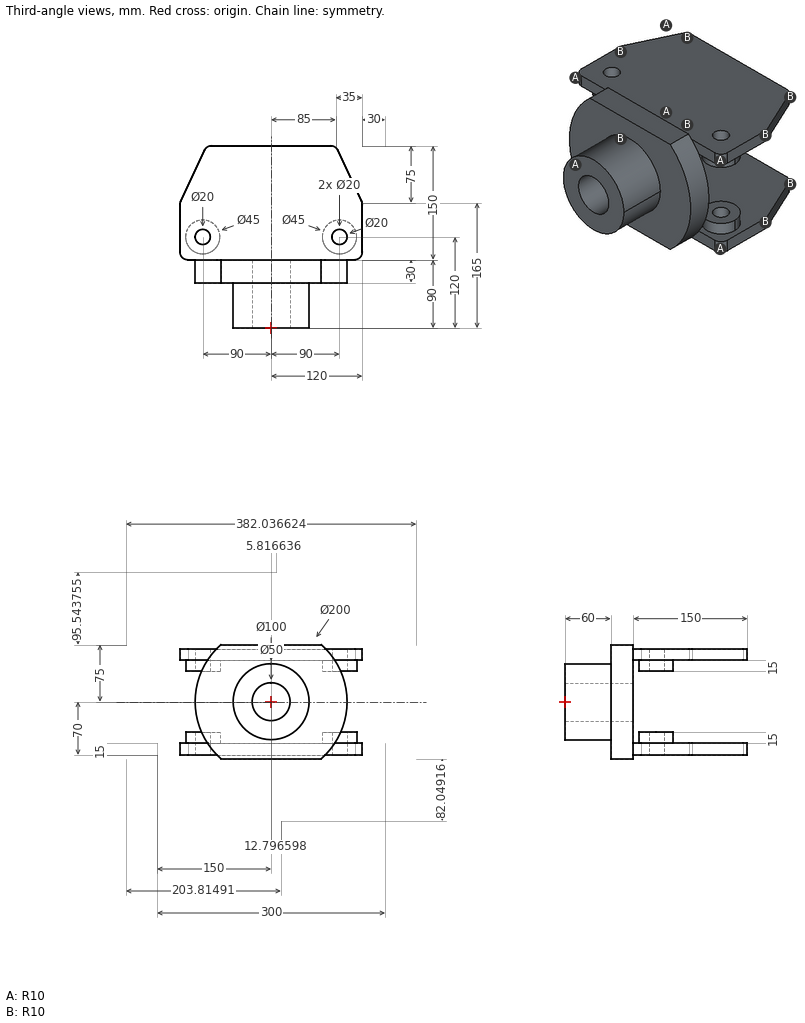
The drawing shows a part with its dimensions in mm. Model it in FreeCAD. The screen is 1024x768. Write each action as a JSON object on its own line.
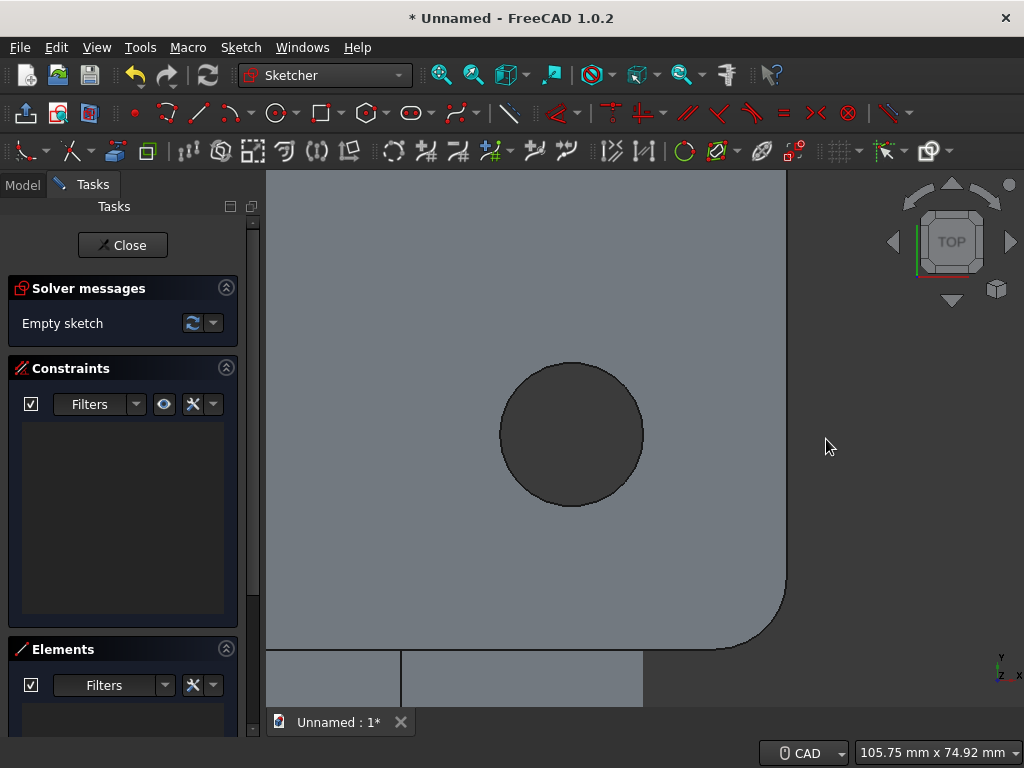
{"action": "left_click", "coordinate": [276, 114]}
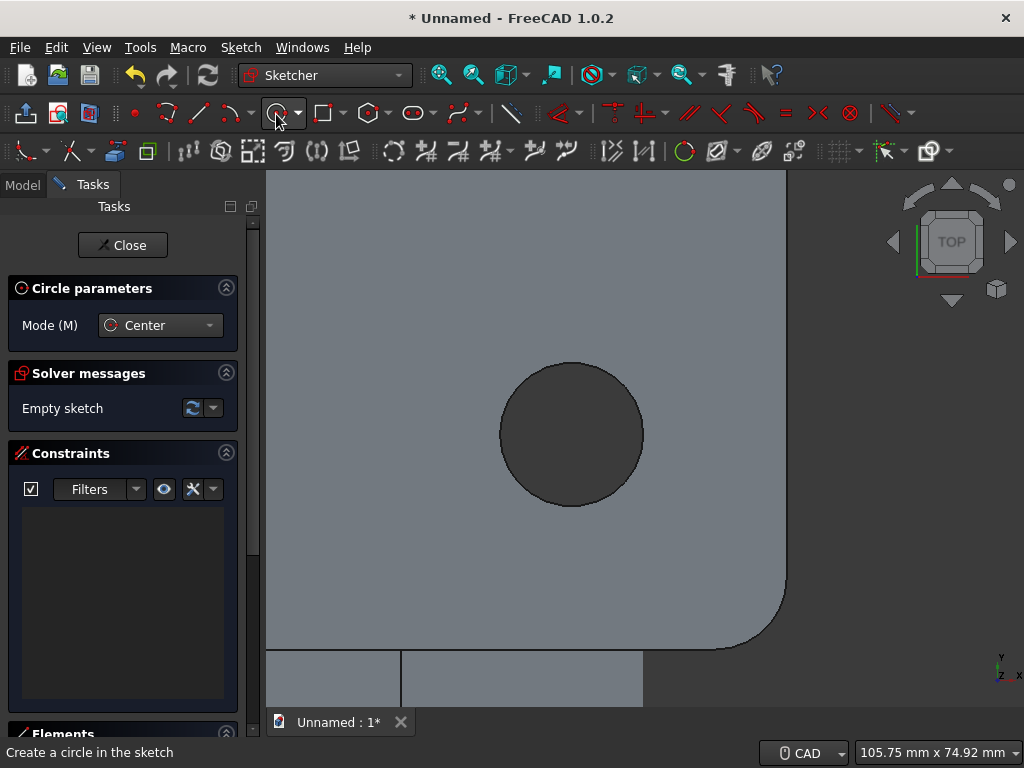
{"action": "left_click", "coordinate": [572, 435]}
{"action": "left_click", "coordinate": [686, 321]}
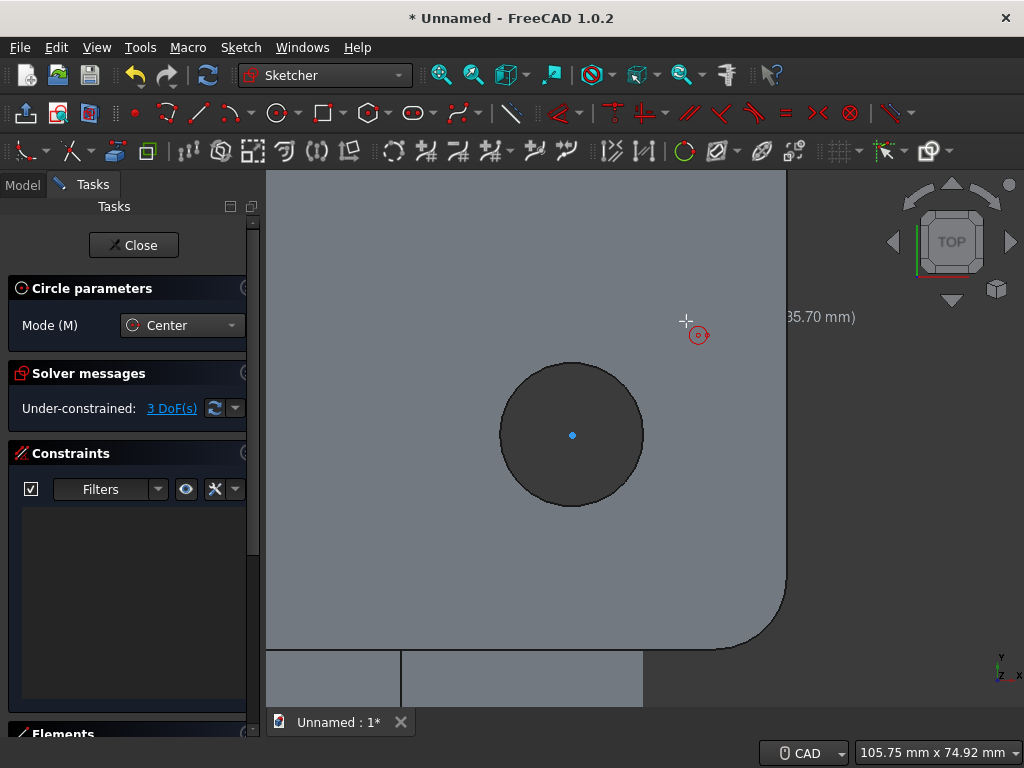
{"action": "left_click", "coordinate": [572, 436]}
{"action": "left_click", "coordinate": [622, 384]}
{"action": "key", "text": "Escape"}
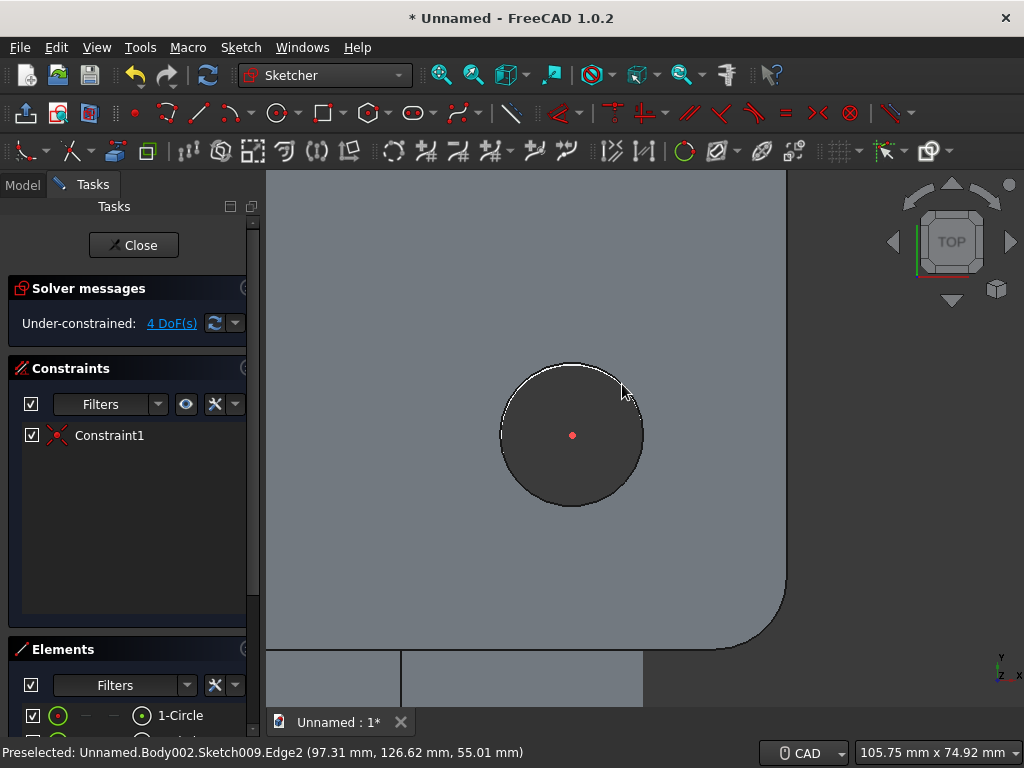
{"action": "left_click", "coordinate": [558, 114]}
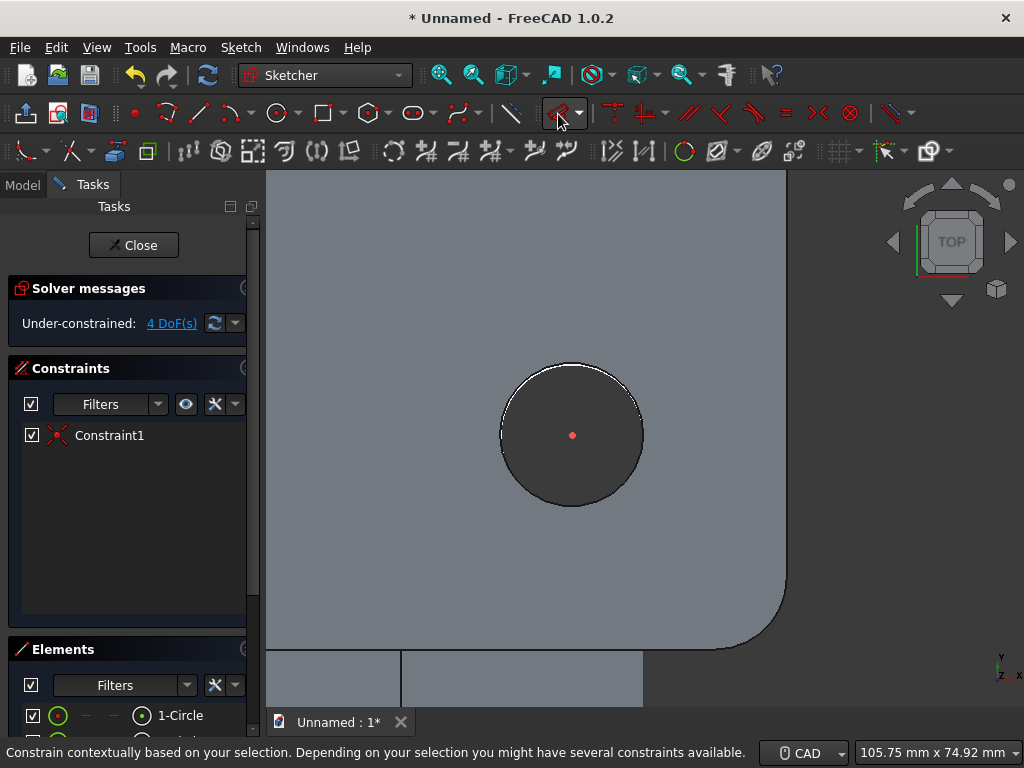
{"action": "left_click", "coordinate": [686, 322]}
{"action": "left_click", "coordinate": [709, 299]}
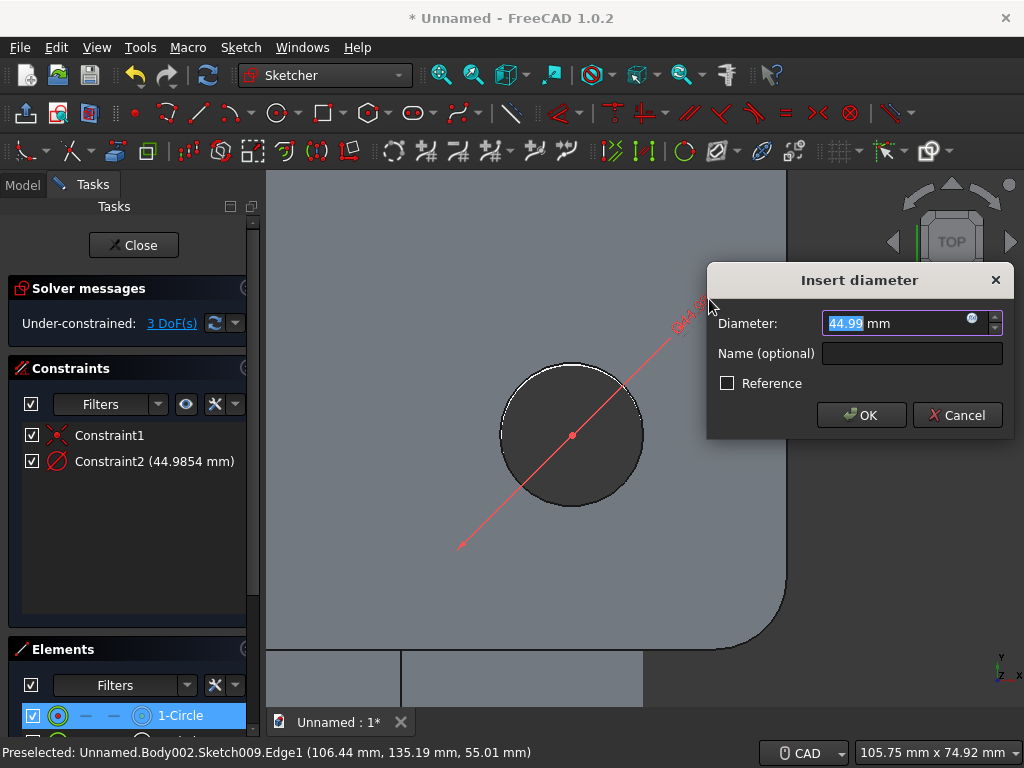
{"action": "type", "text": "45"}
{"action": "key", "text": "Return"}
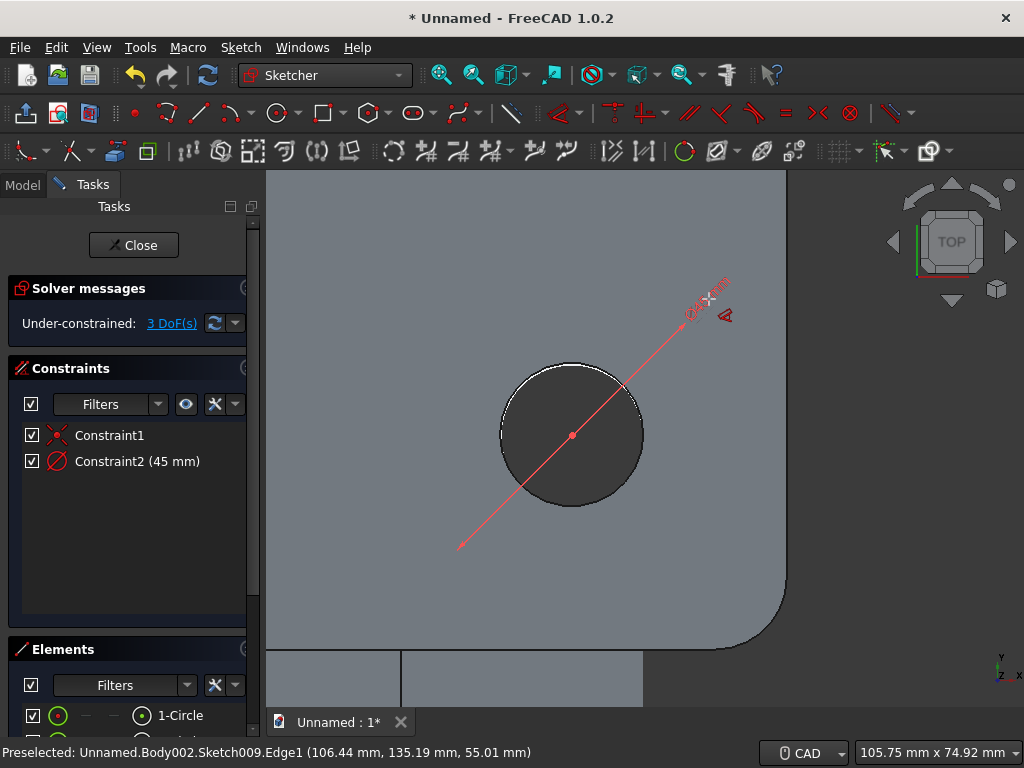
{"action": "left_click", "coordinate": [622, 385]}
{"action": "left_click", "coordinate": [644, 362]}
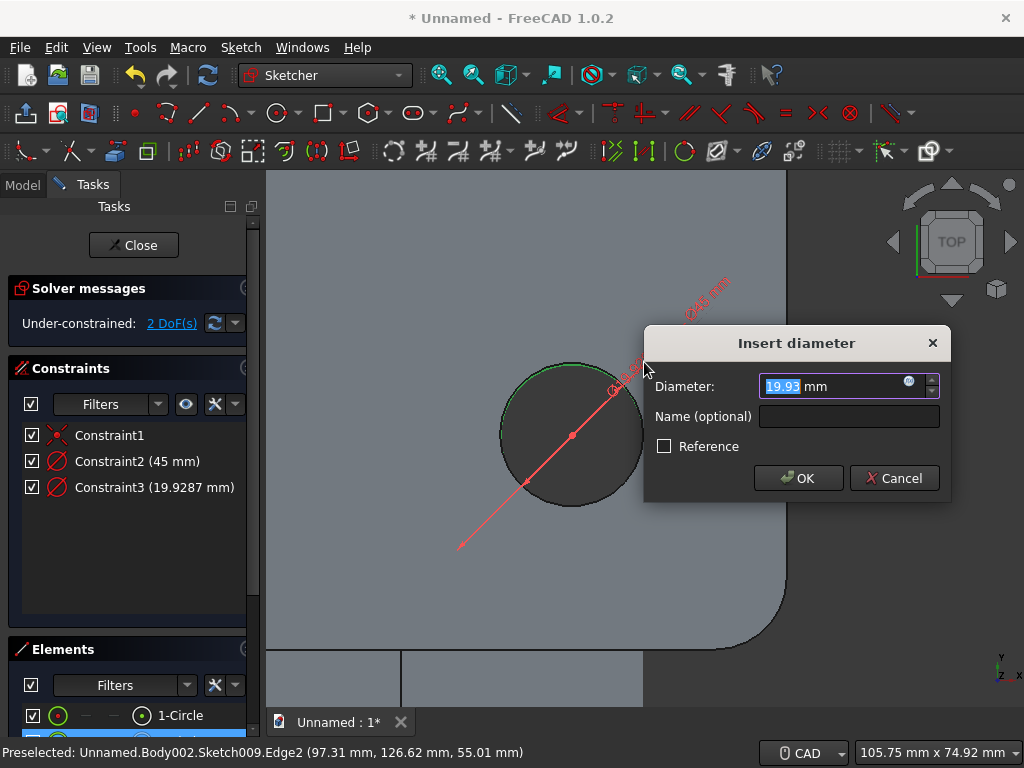
{"action": "type", "text": "20"}
{"action": "key", "text": "Return"}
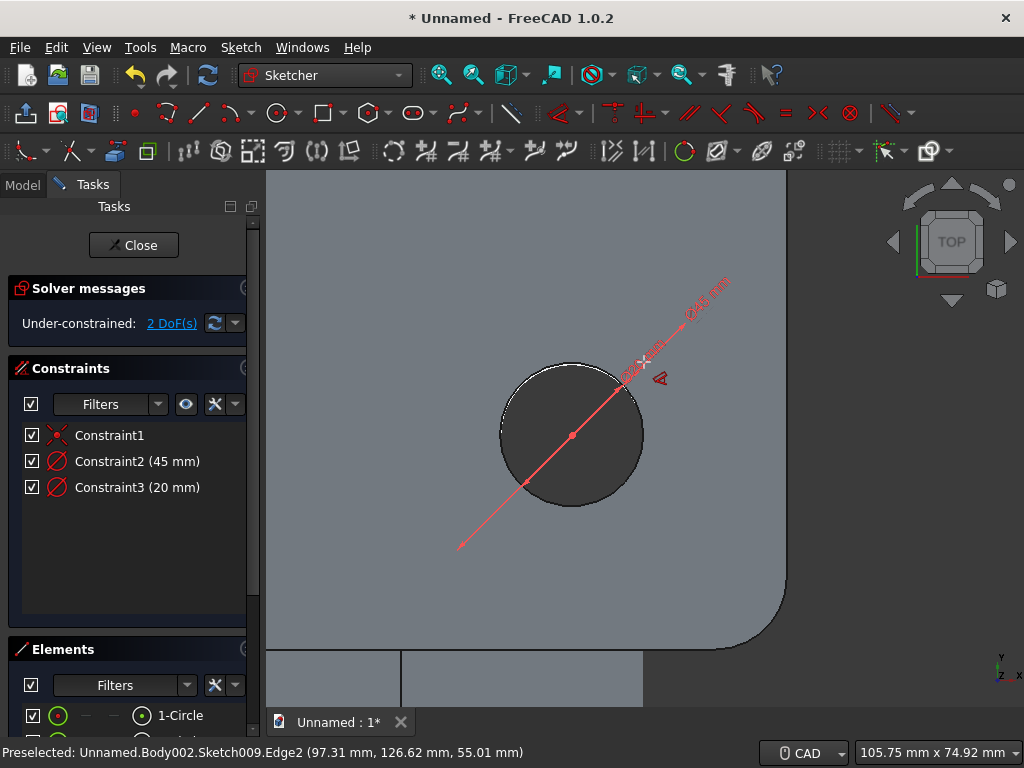
{"action": "left_click", "coordinate": [572, 436]}
{"action": "left_click", "coordinate": [433, 402]}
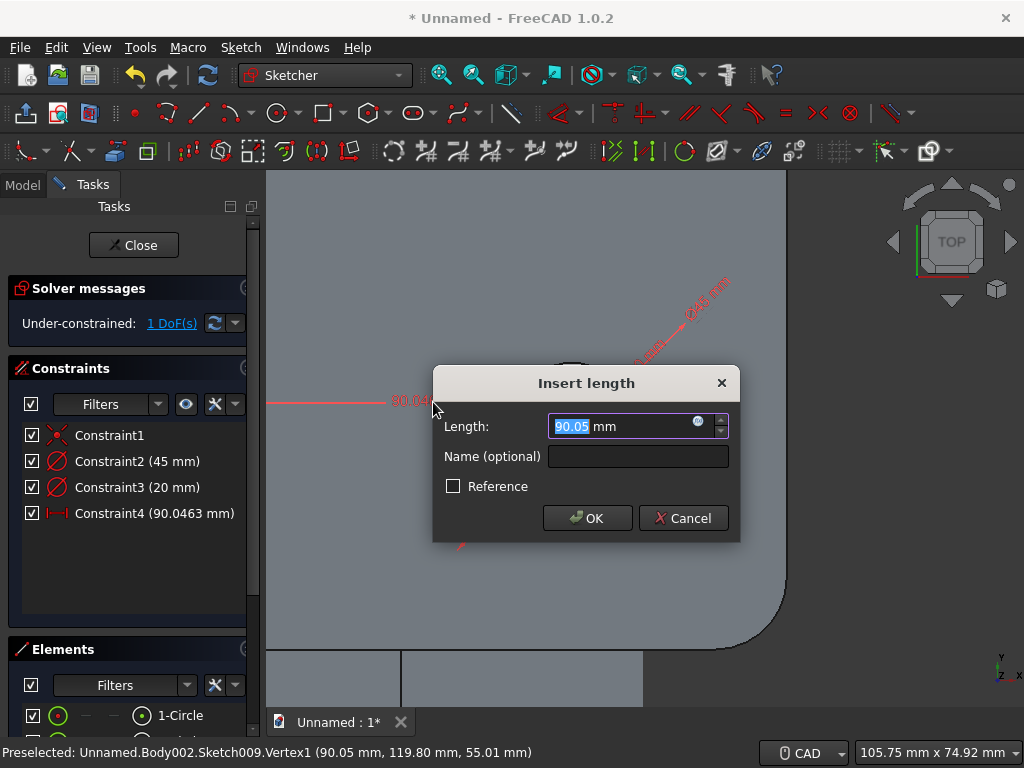
{"action": "type", "text": "90"}
{"action": "key", "text": "Return"}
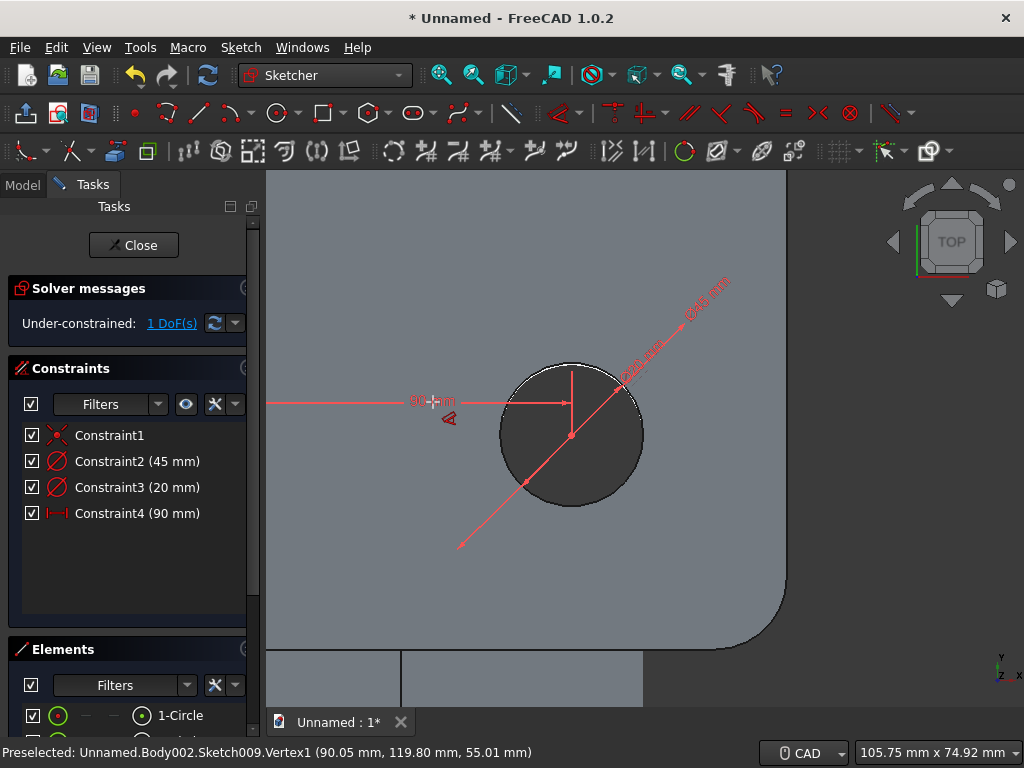
{"action": "left_click", "coordinate": [572, 436]}
{"action": "left_click", "coordinate": [606, 558]}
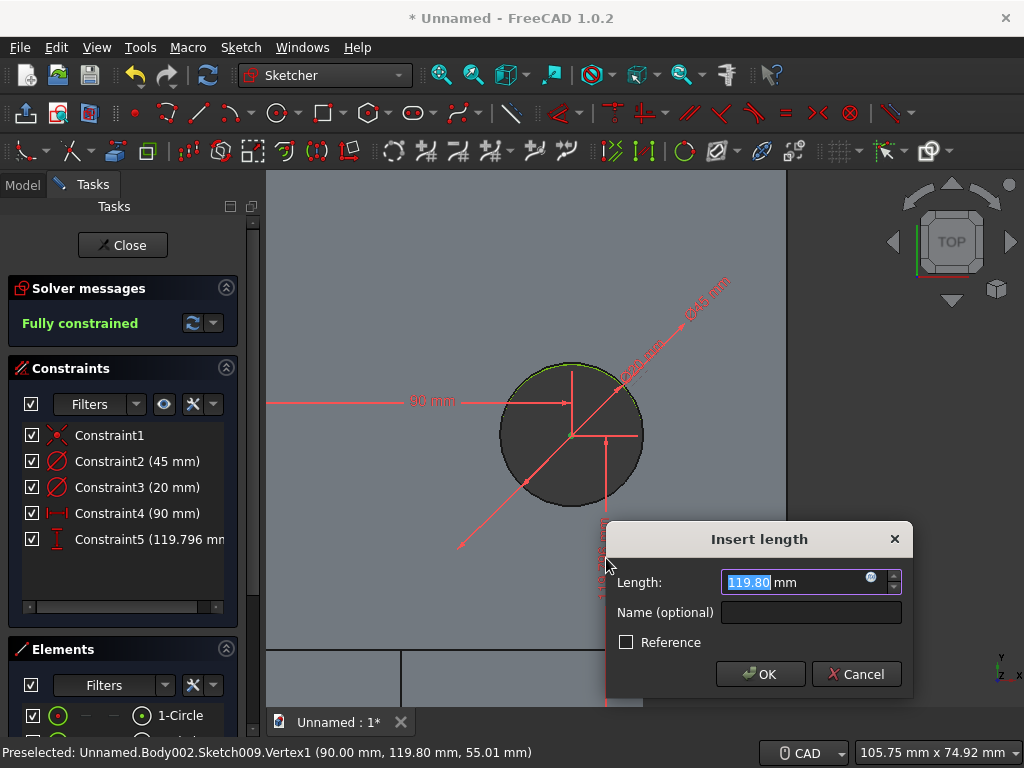
{"action": "type", "text": "120"}
{"action": "key", "text": "Return"}
{"action": "key", "text": "Escape"}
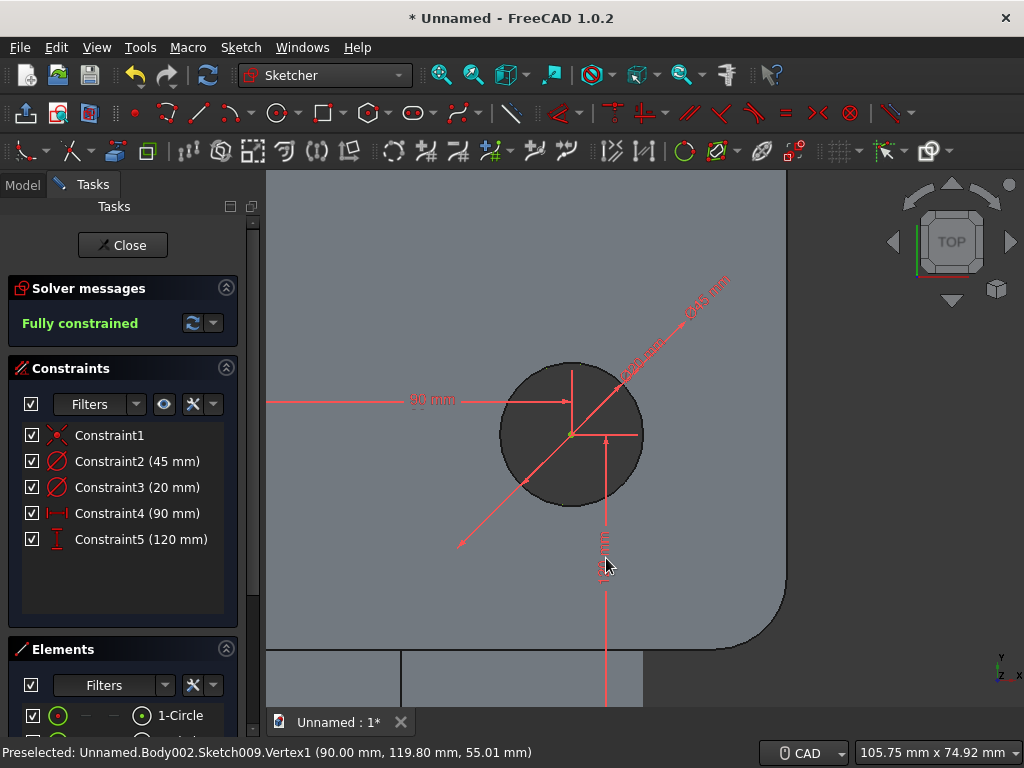
{"action": "left_click", "coordinate": [123, 245]}